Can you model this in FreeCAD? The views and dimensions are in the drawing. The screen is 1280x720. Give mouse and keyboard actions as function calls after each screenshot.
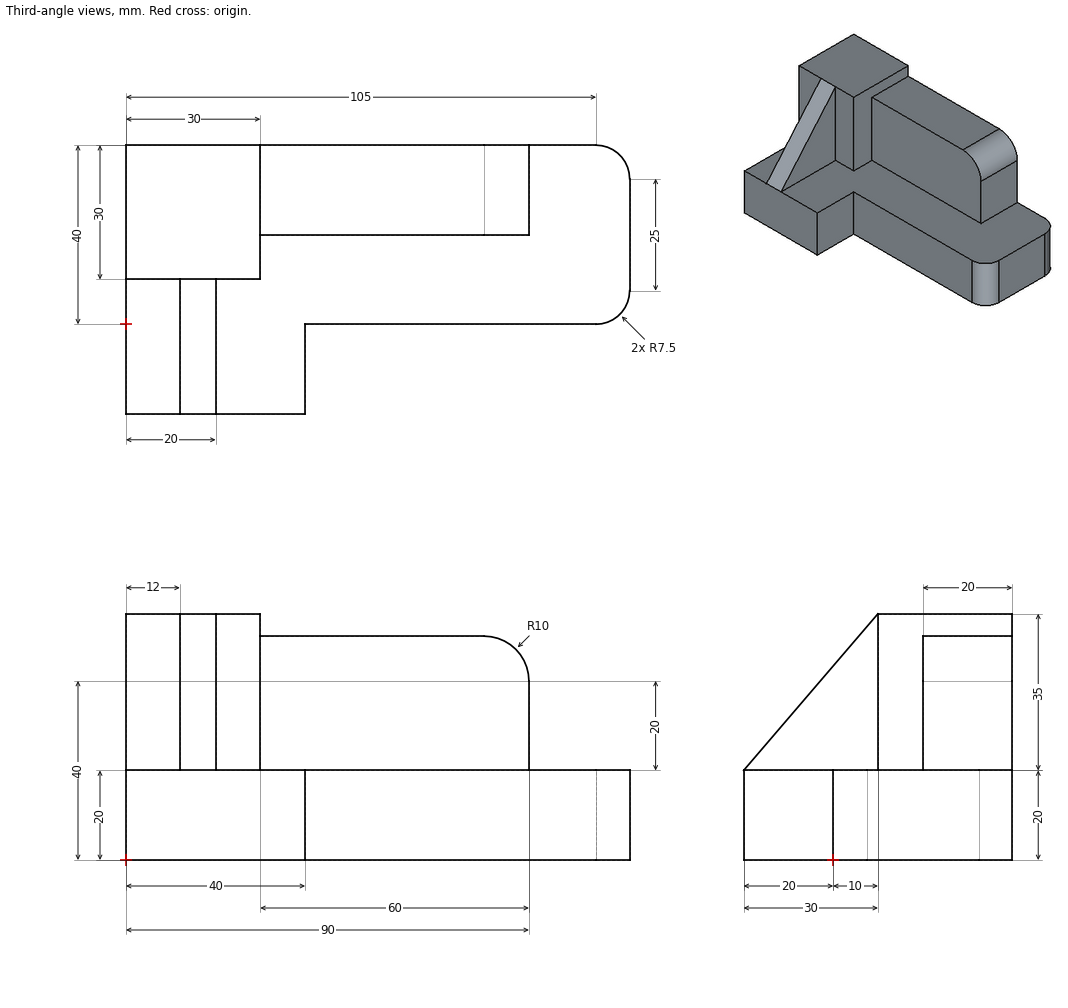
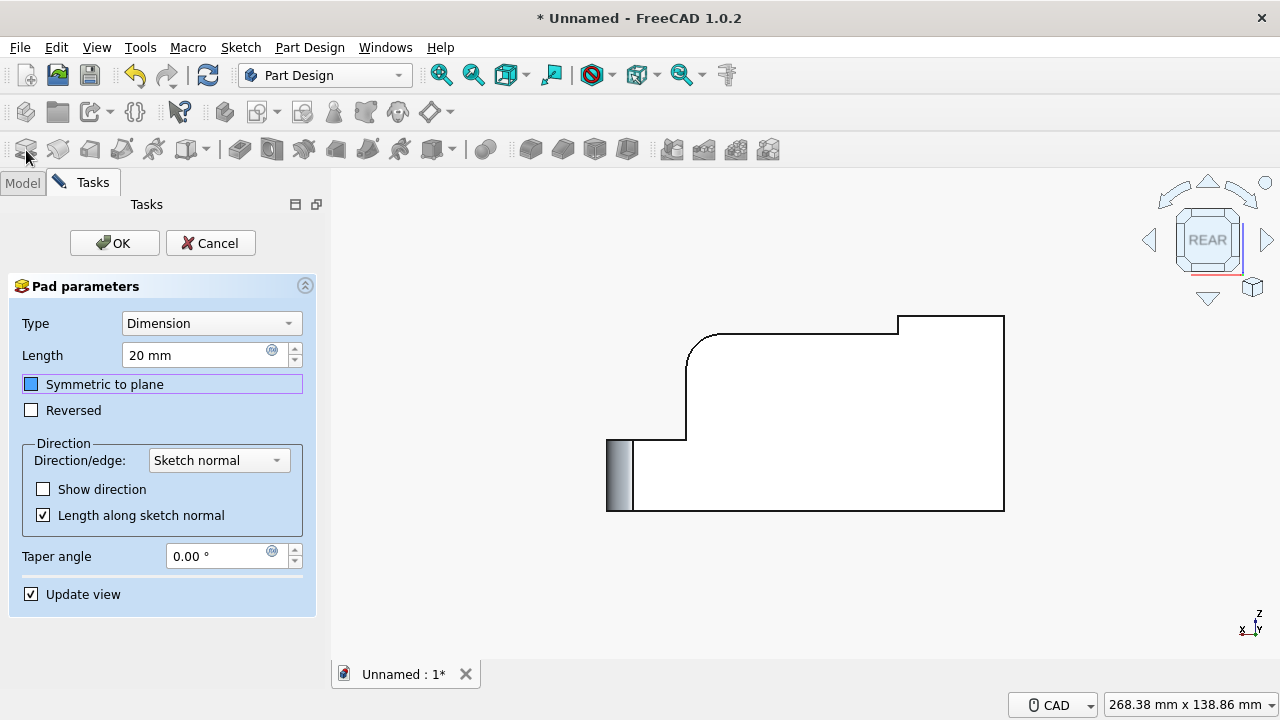
click(115, 243)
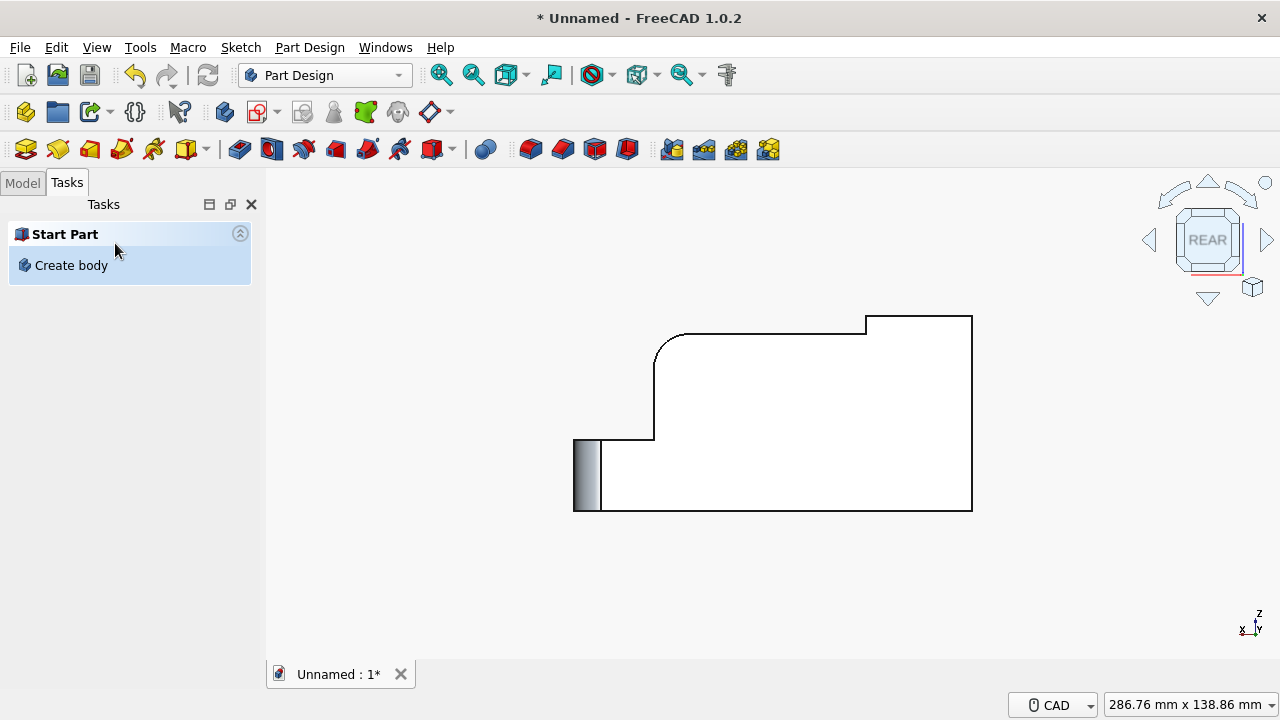
key(v)
key(f)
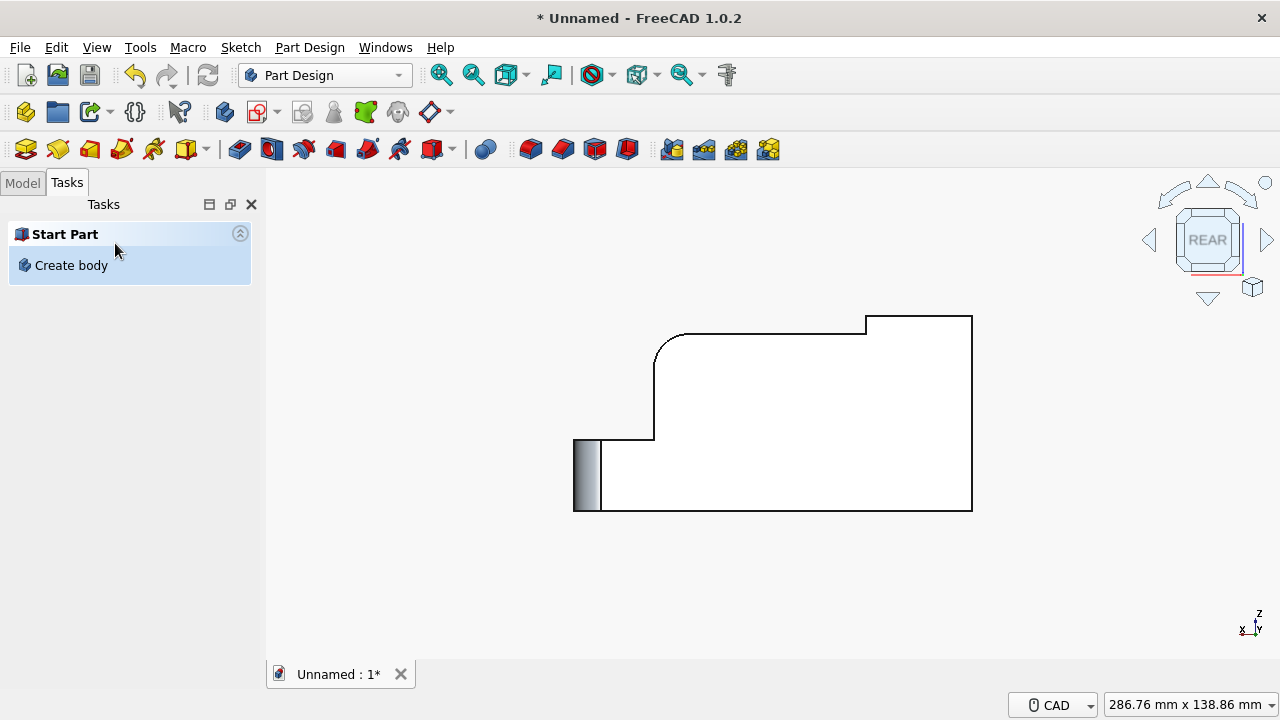
key(6)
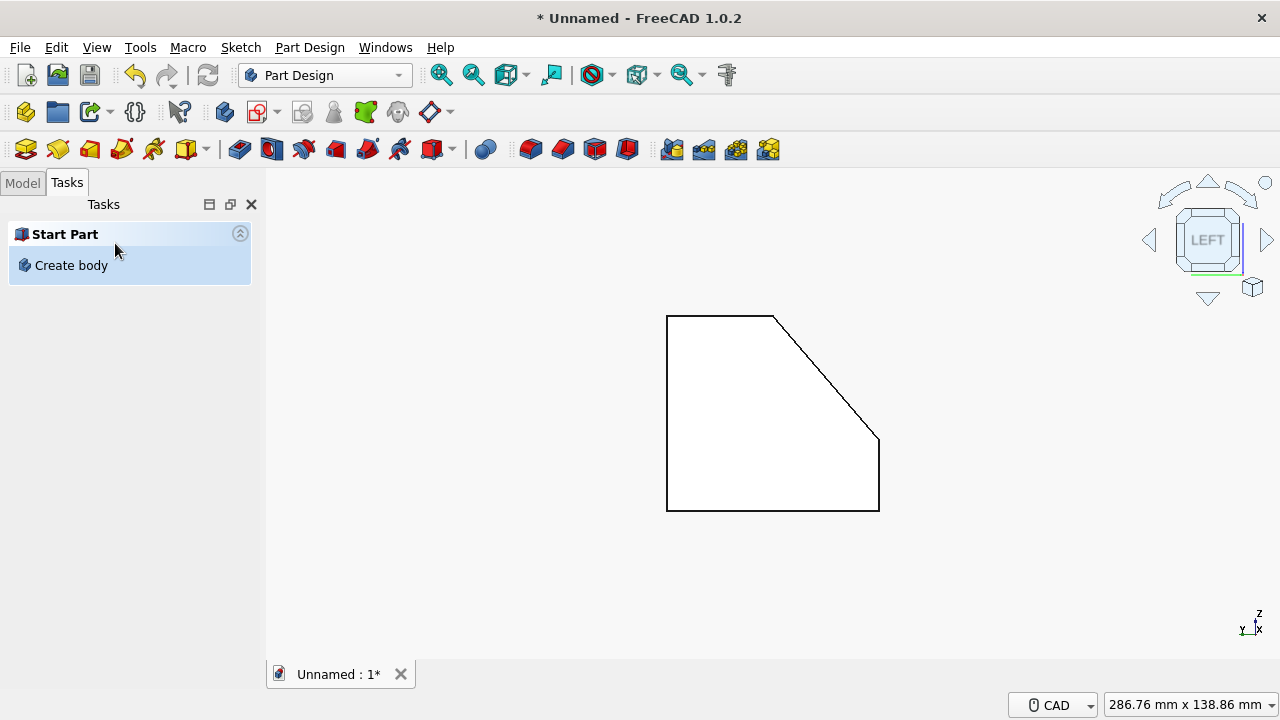
key(v)
key(f)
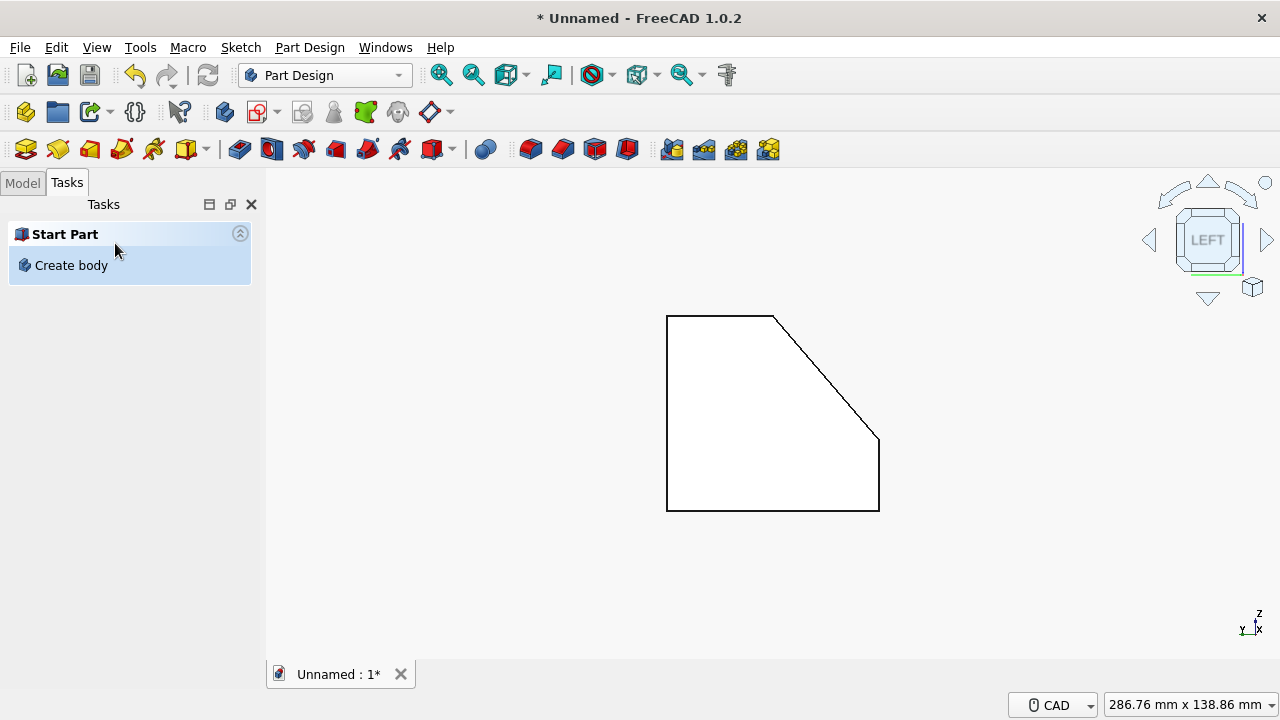
click(743, 412)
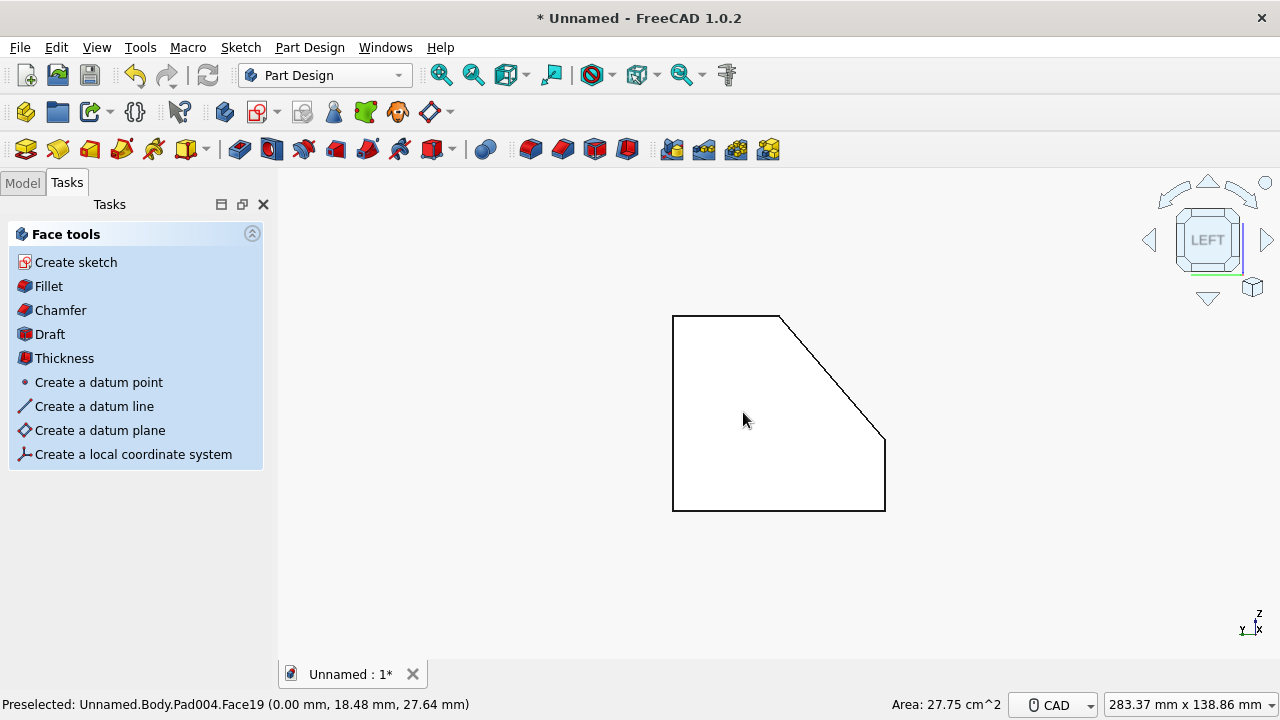
click(258, 112)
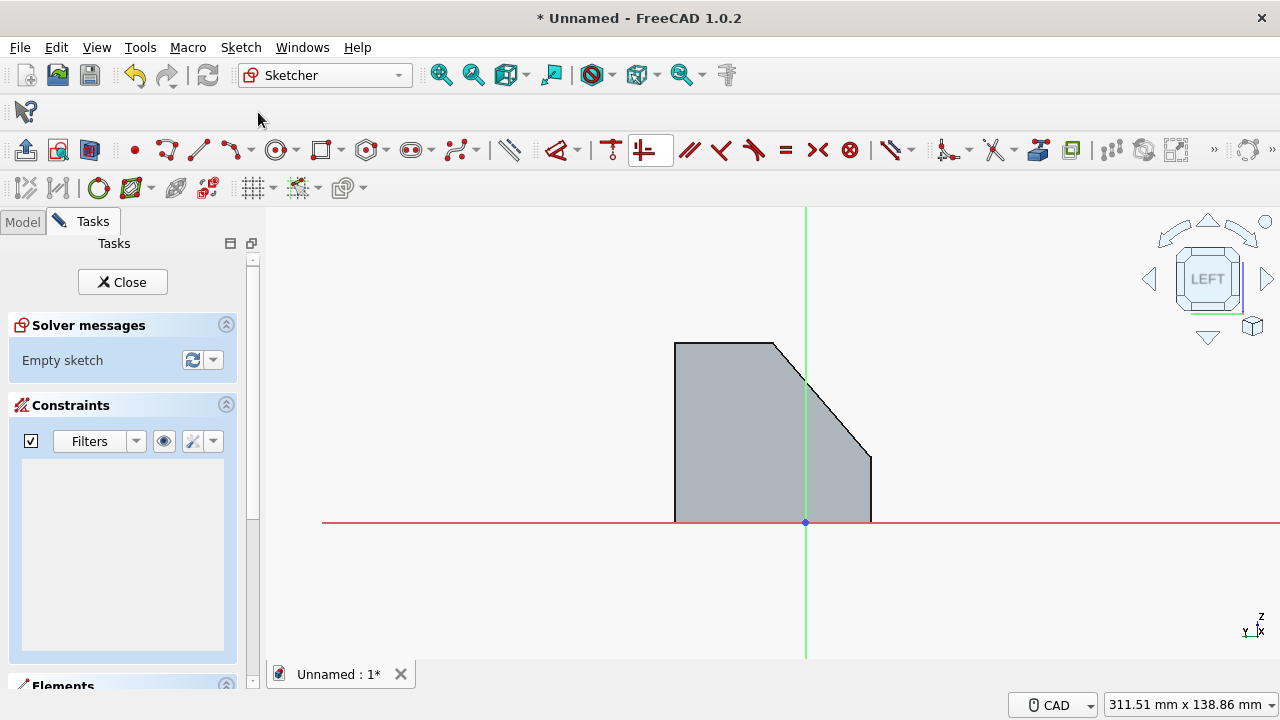
scroll(1060, 433, up, 2)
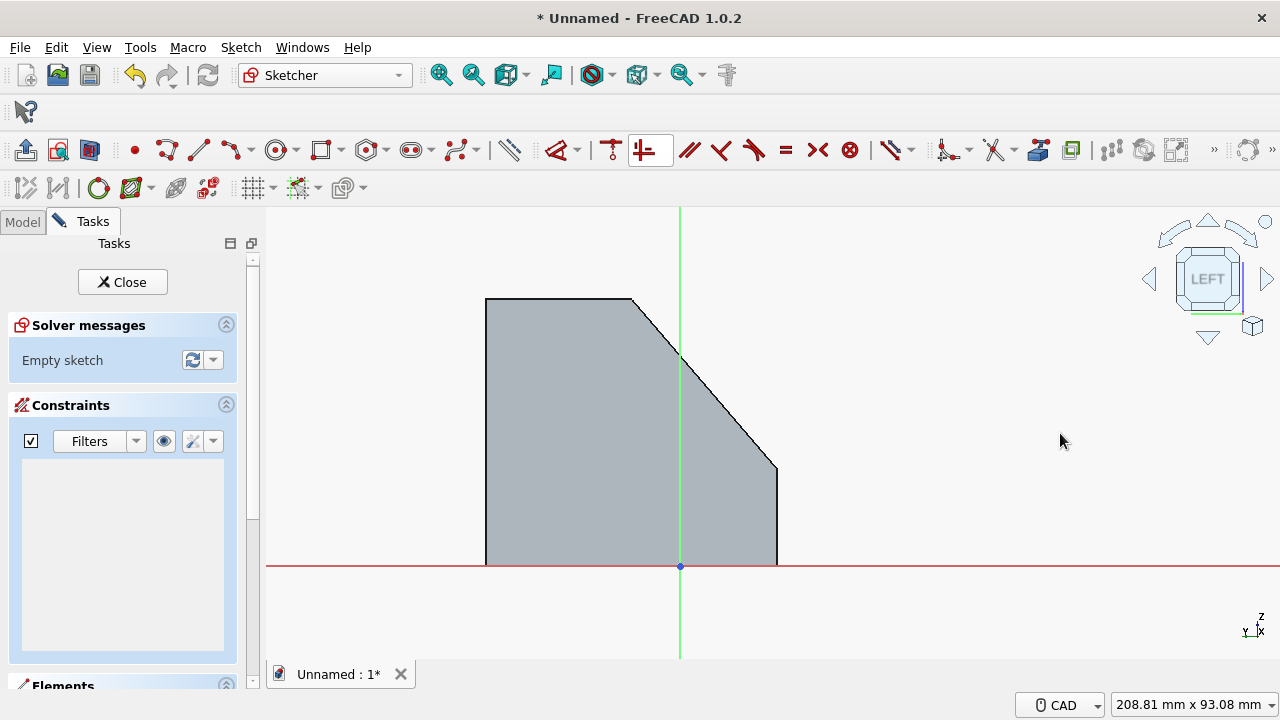
key(g)
key(m)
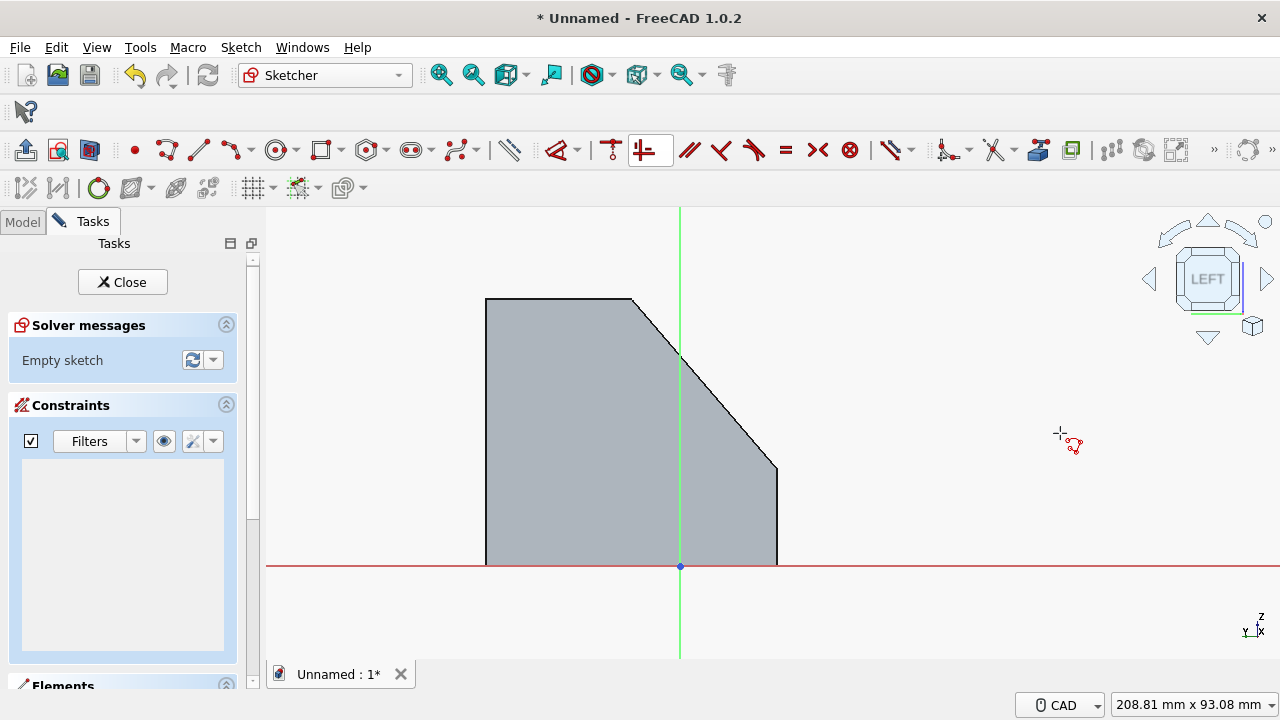
click(631, 469)
click(777, 469)
click(631, 299)
click(631, 470)
key(Escape)
key(Escape)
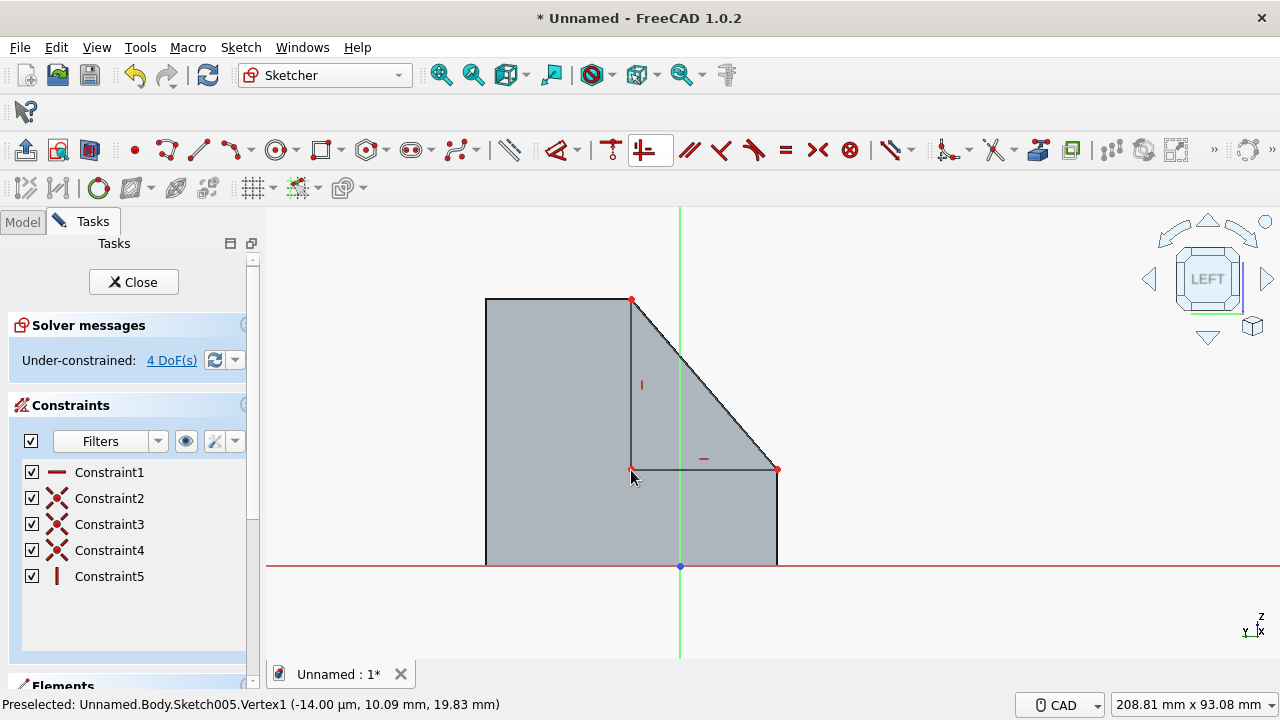
key(d)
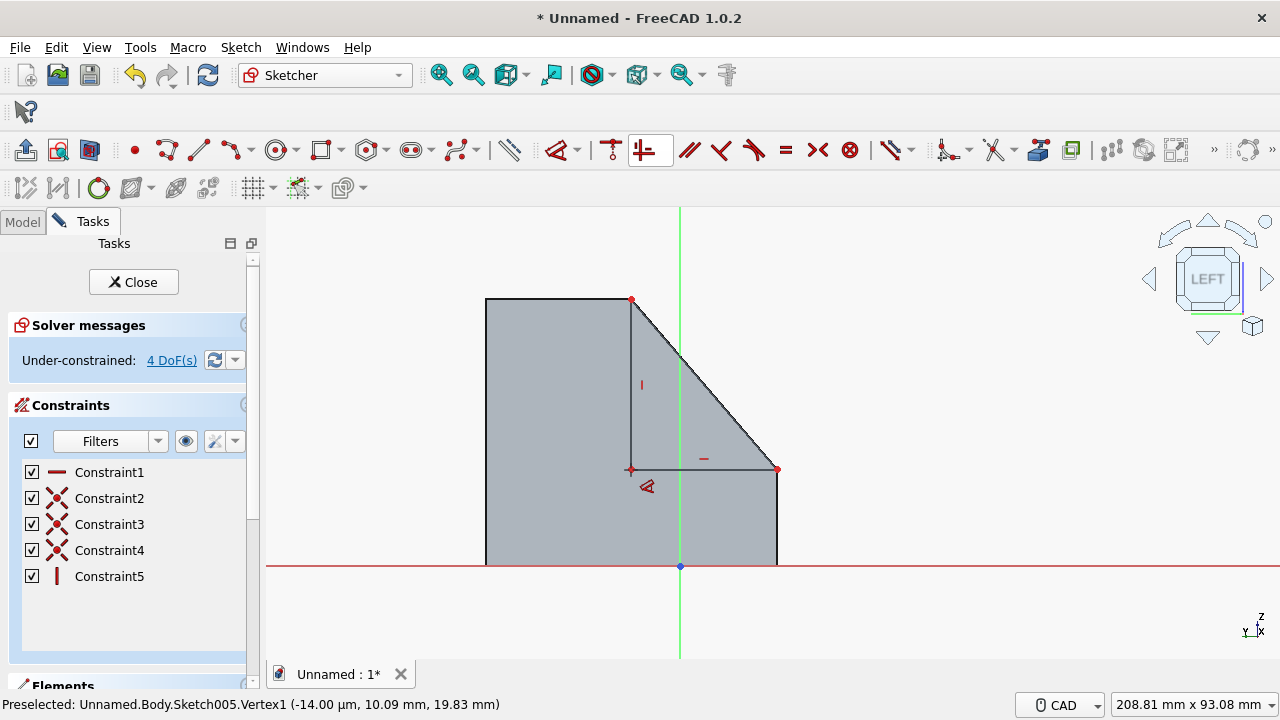
click(733, 470)
click(704, 504)